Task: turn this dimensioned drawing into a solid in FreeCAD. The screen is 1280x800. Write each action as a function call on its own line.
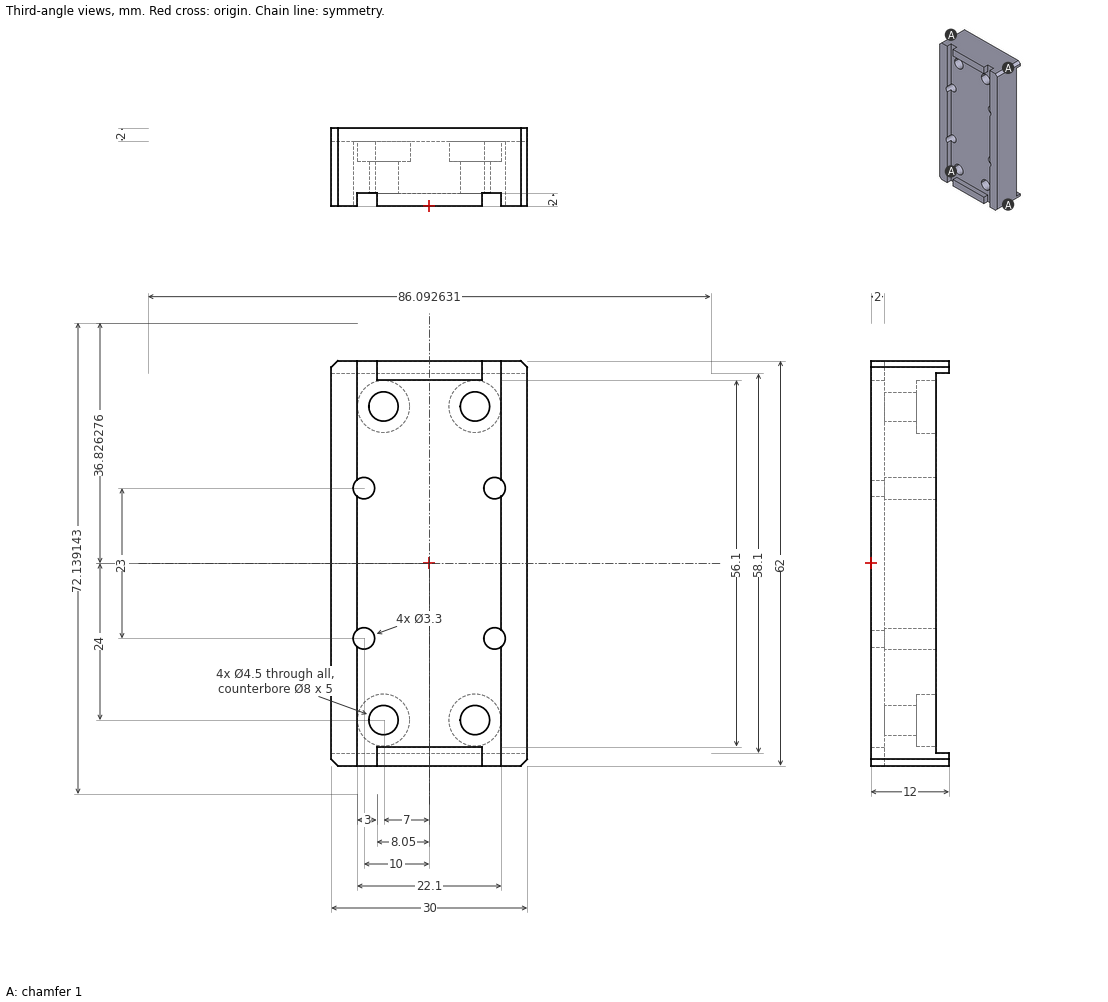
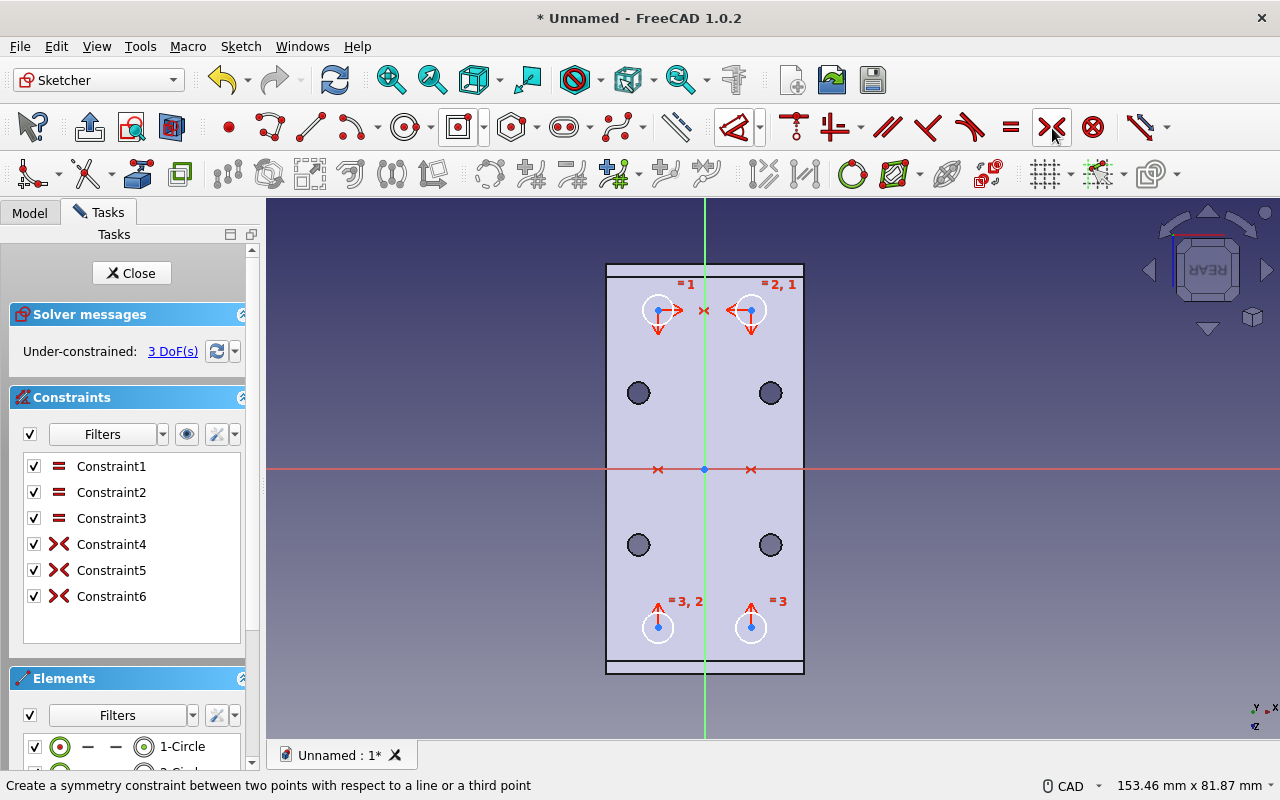
scroll(669, 299, up, 2)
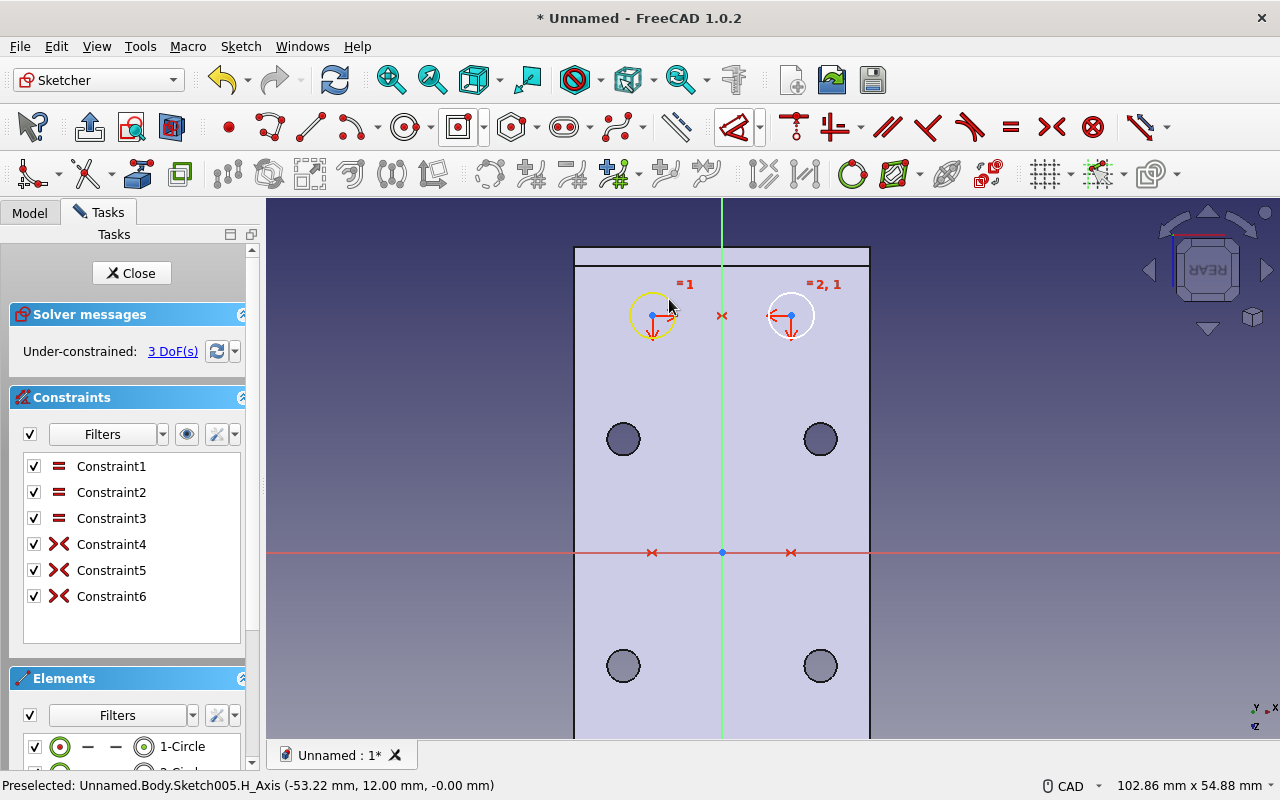
click(669, 300)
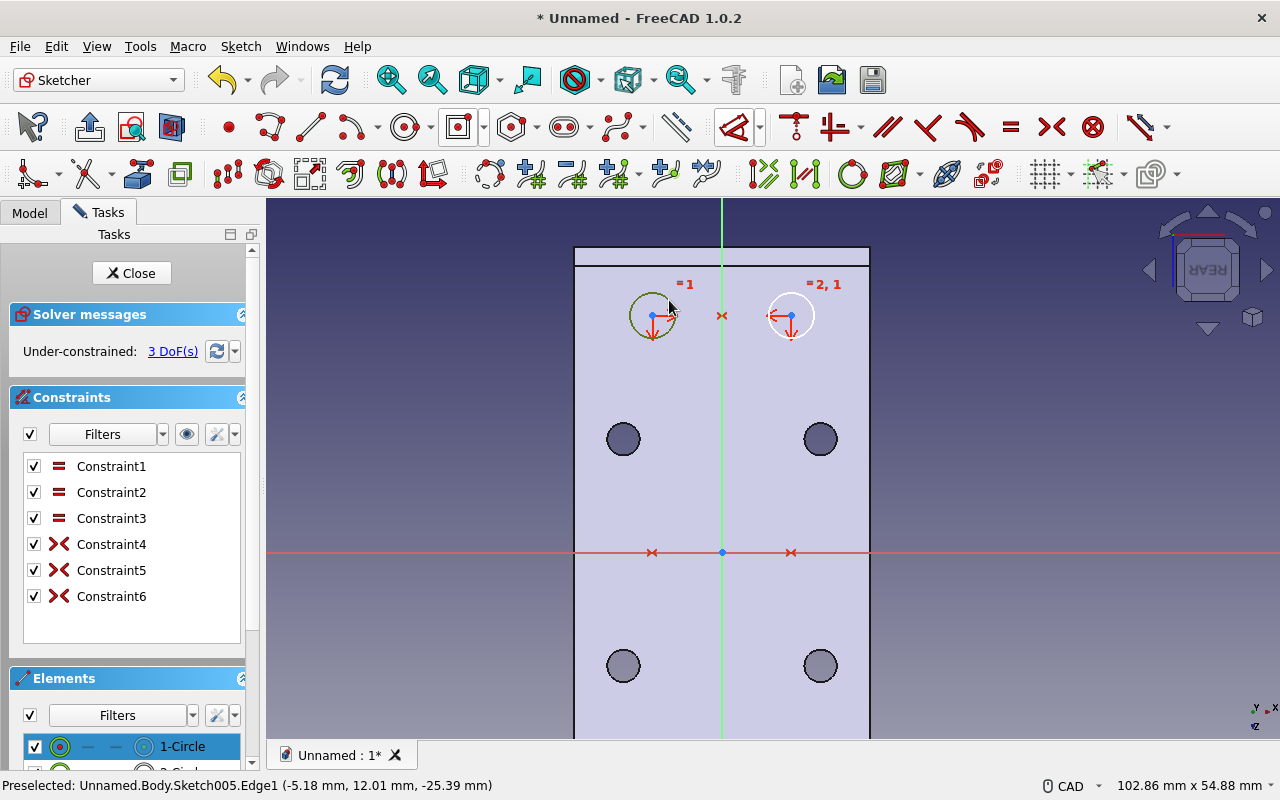
click(760, 128)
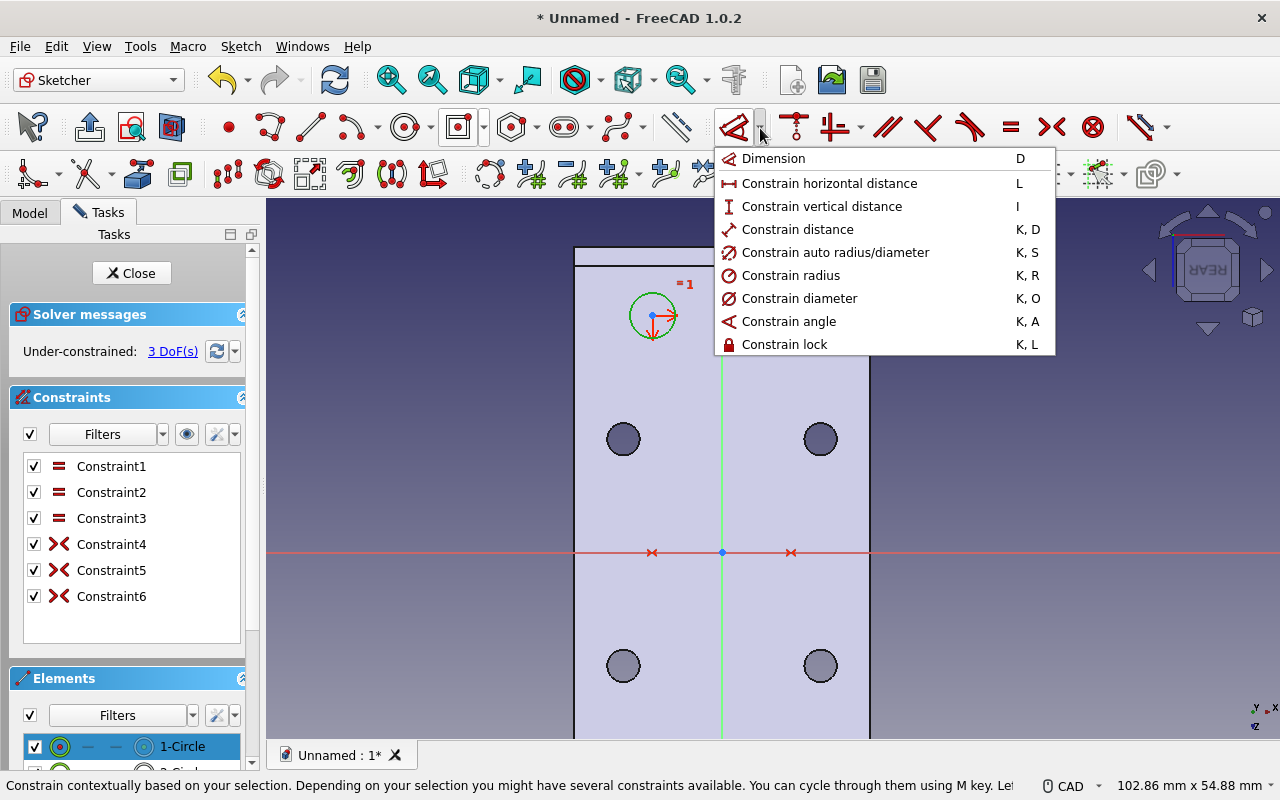
click(885, 298)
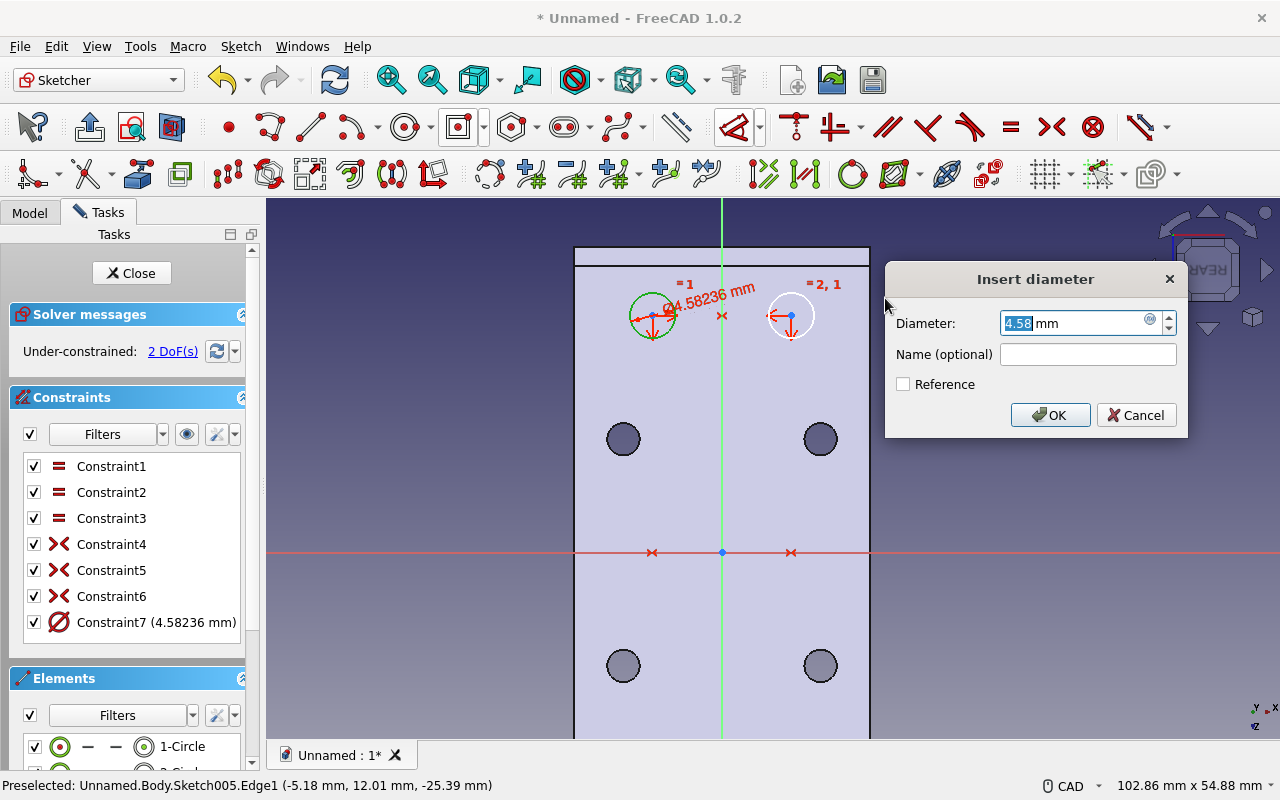
text(4.5)
key(Return)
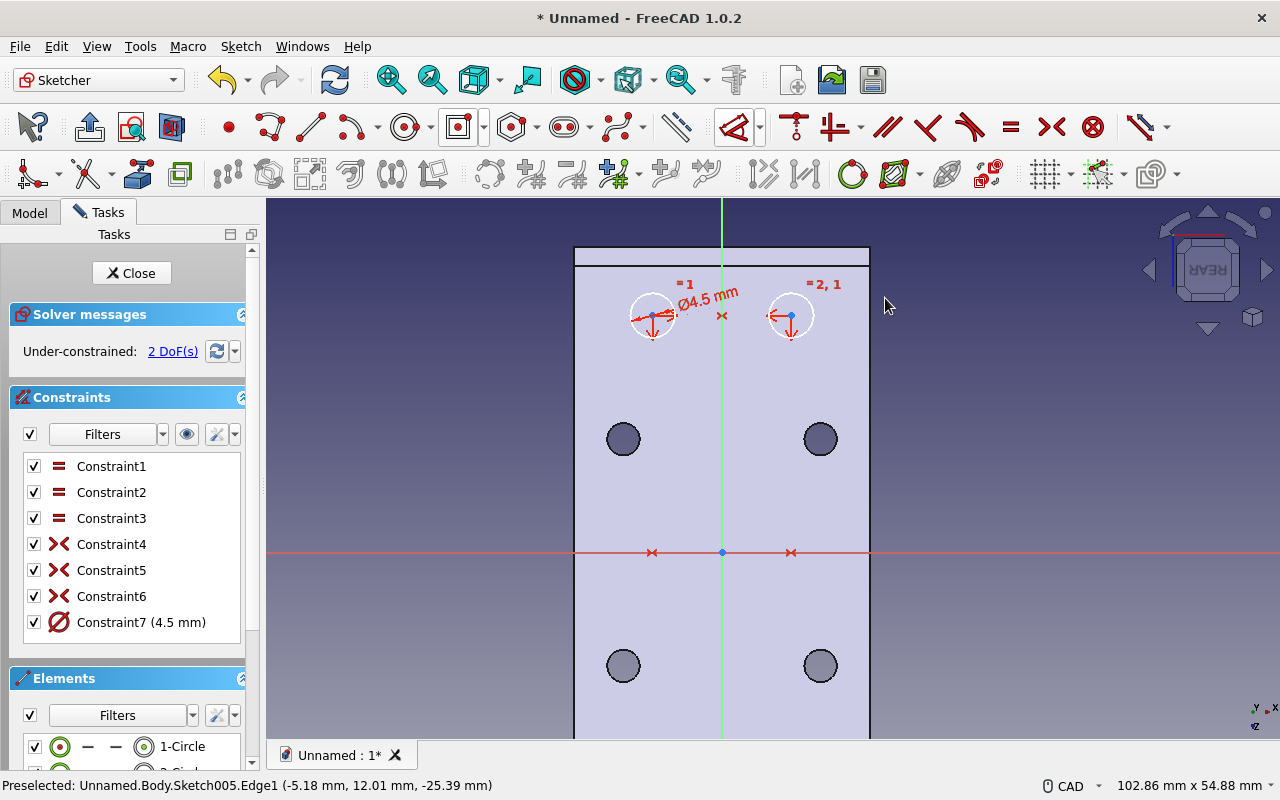
click(653, 316)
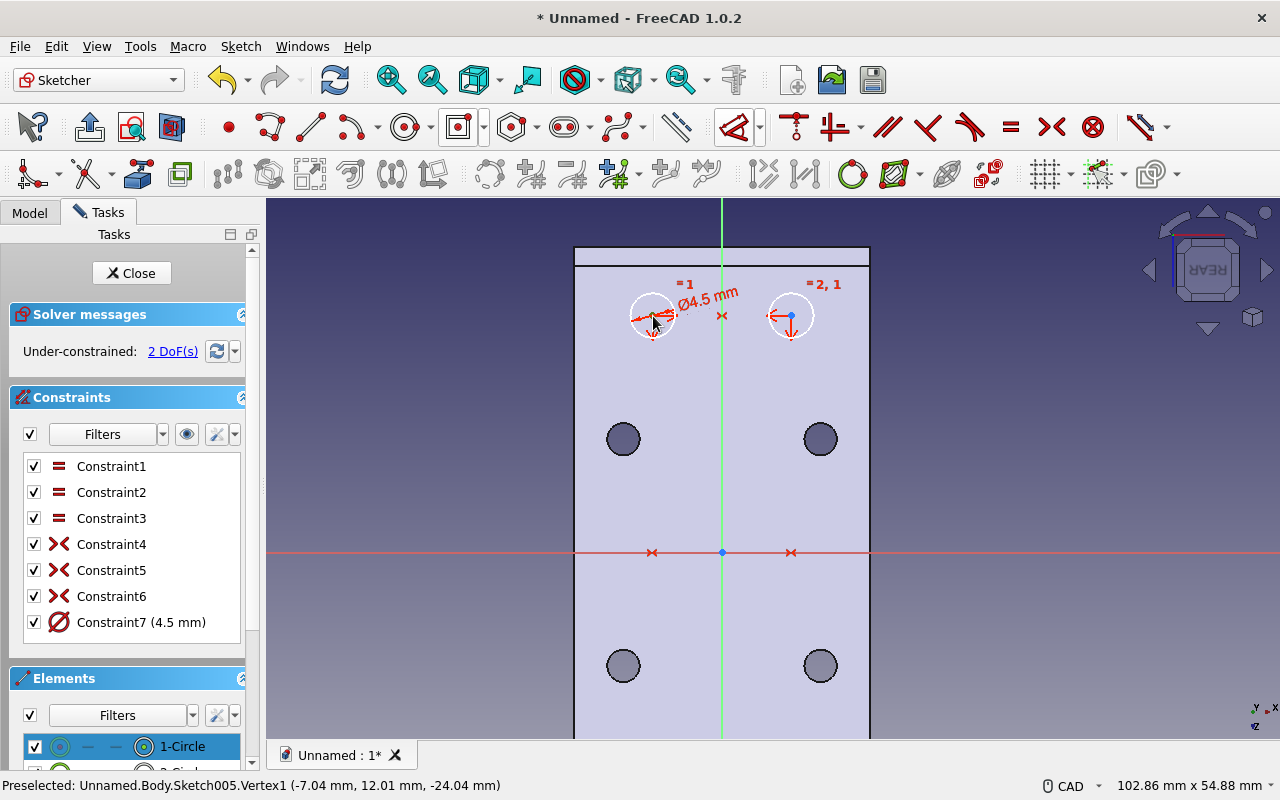
click(760, 128)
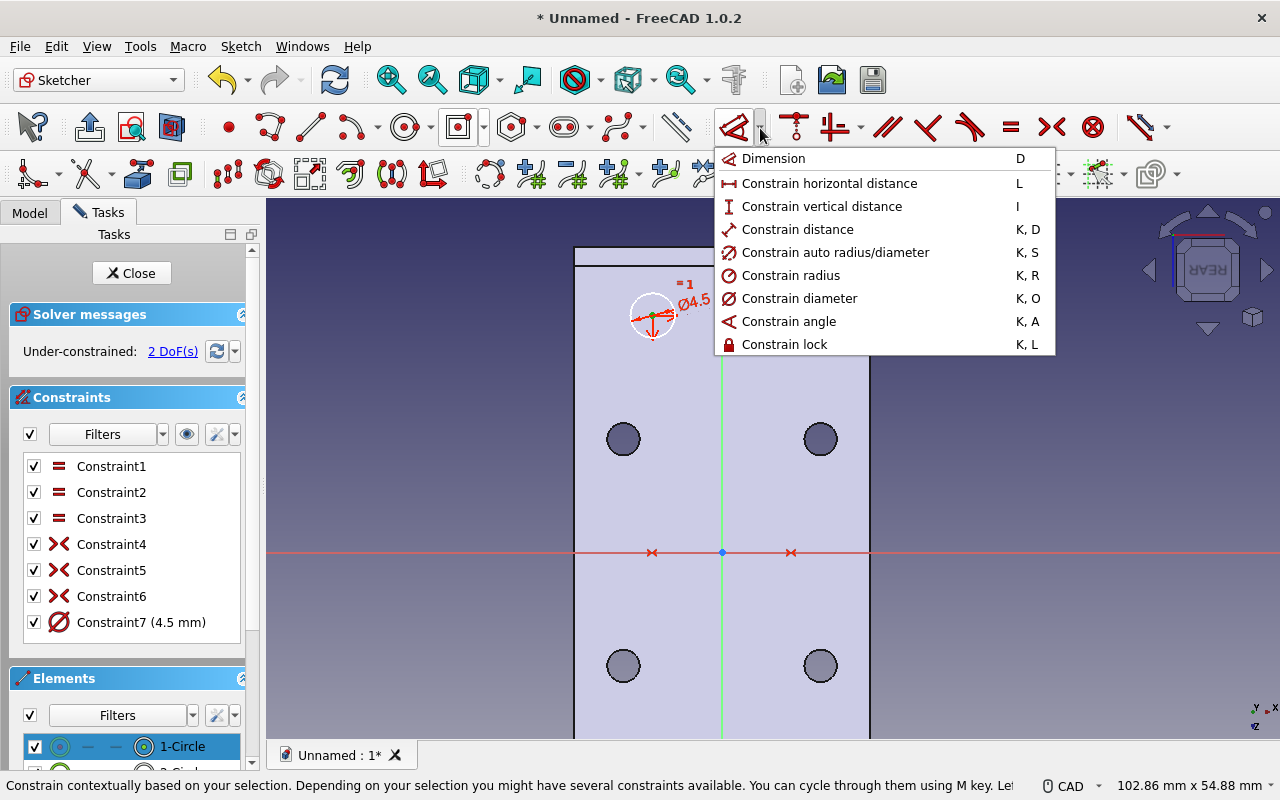
click(885, 184)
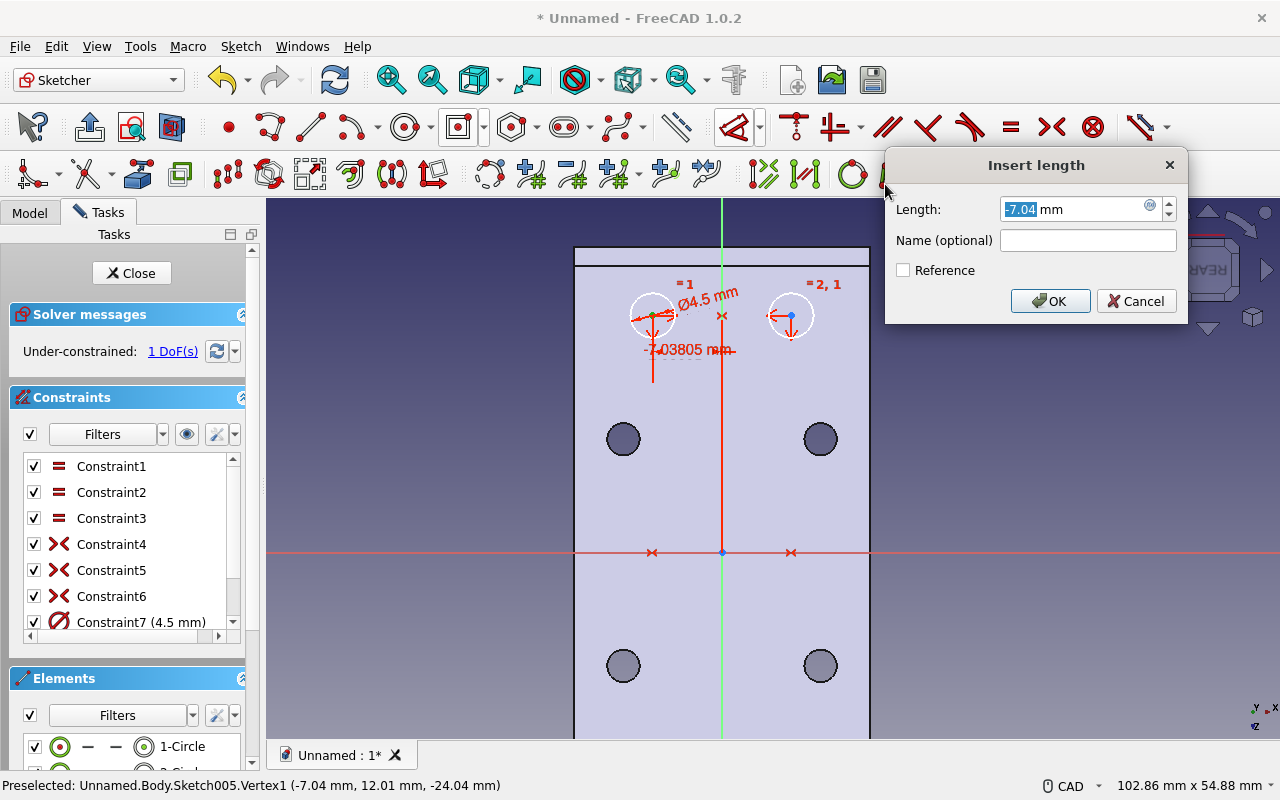
text(-7)
key(Return)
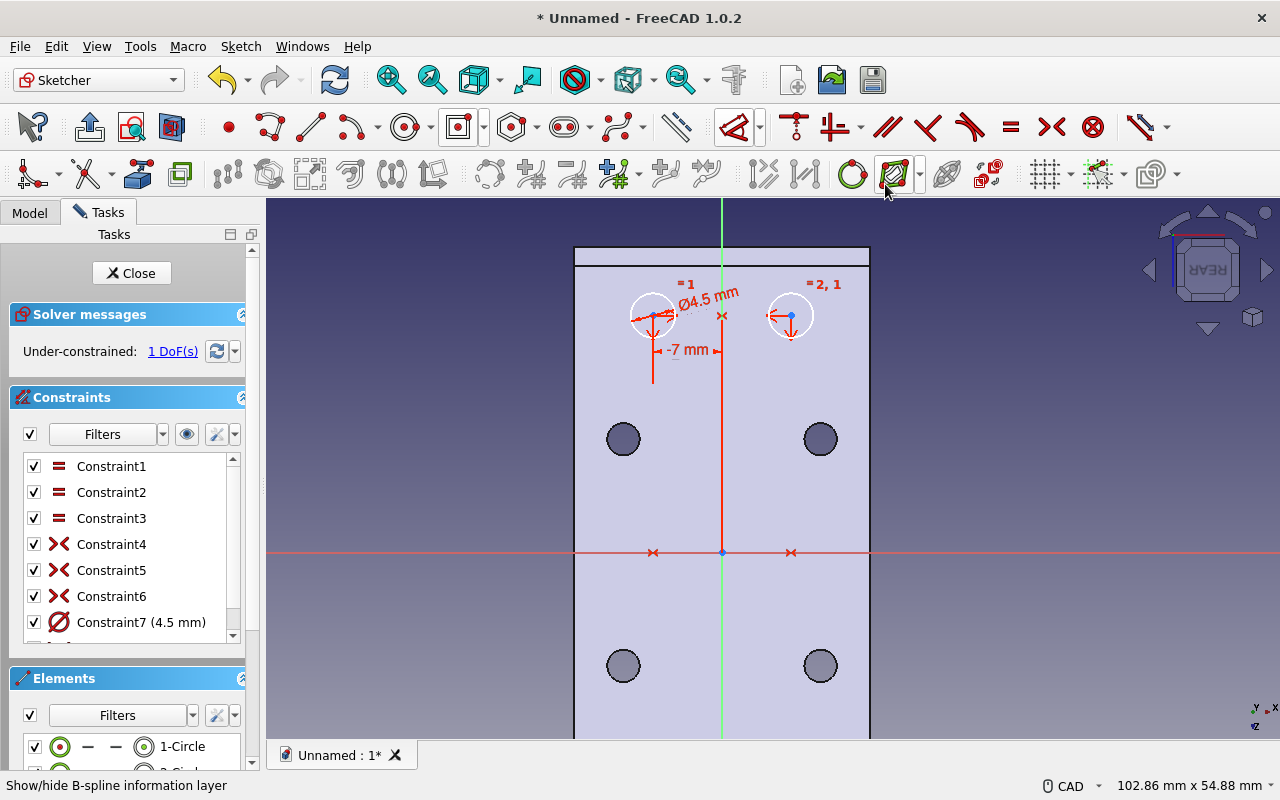
click(653, 316)